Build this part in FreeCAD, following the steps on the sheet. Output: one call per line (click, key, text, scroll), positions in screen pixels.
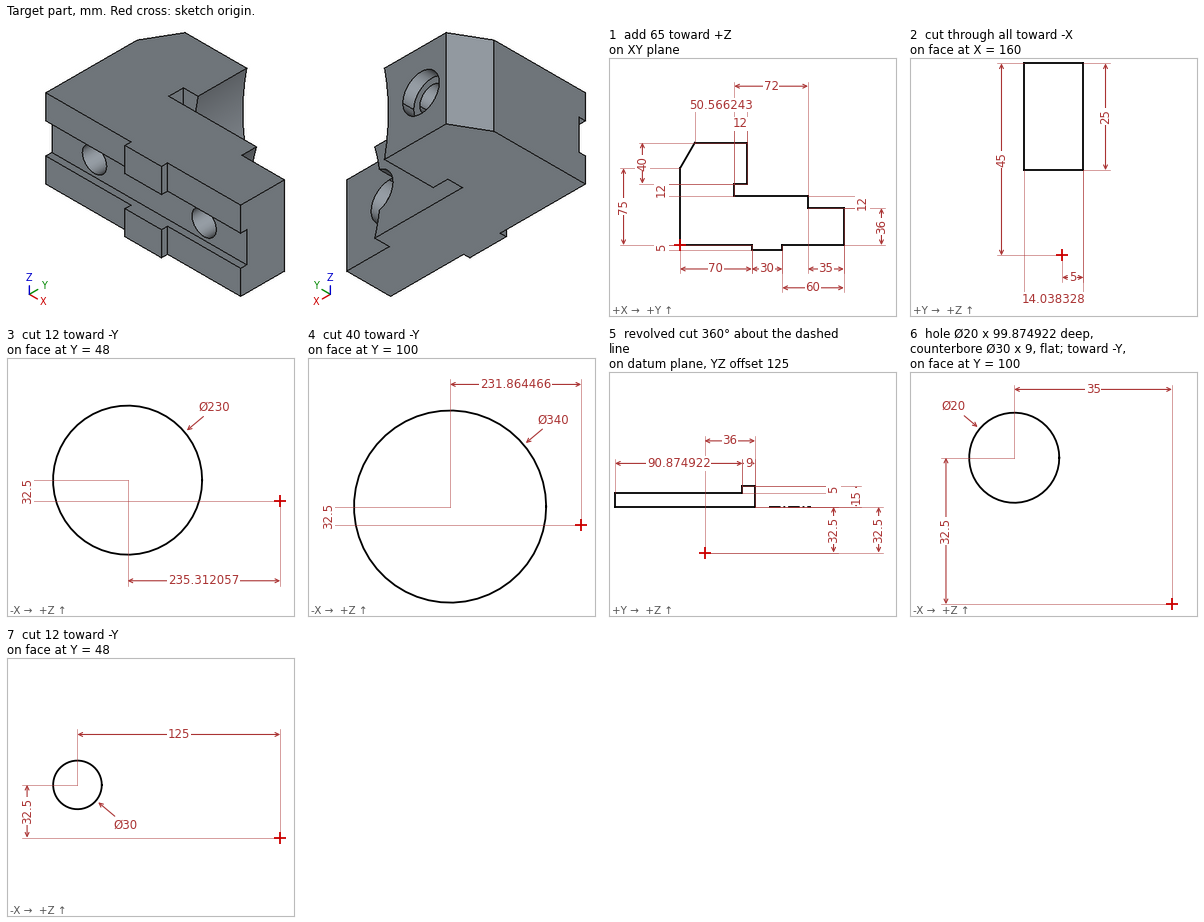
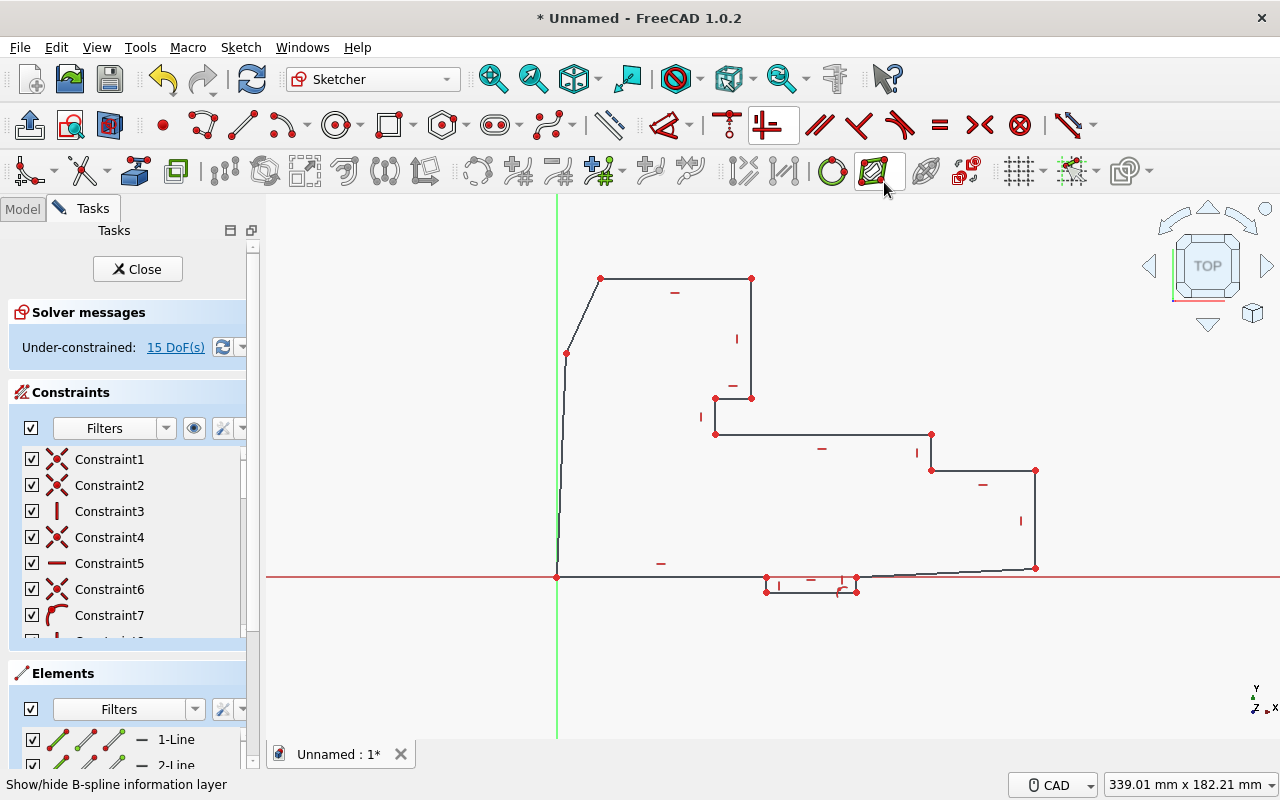
click(910, 575)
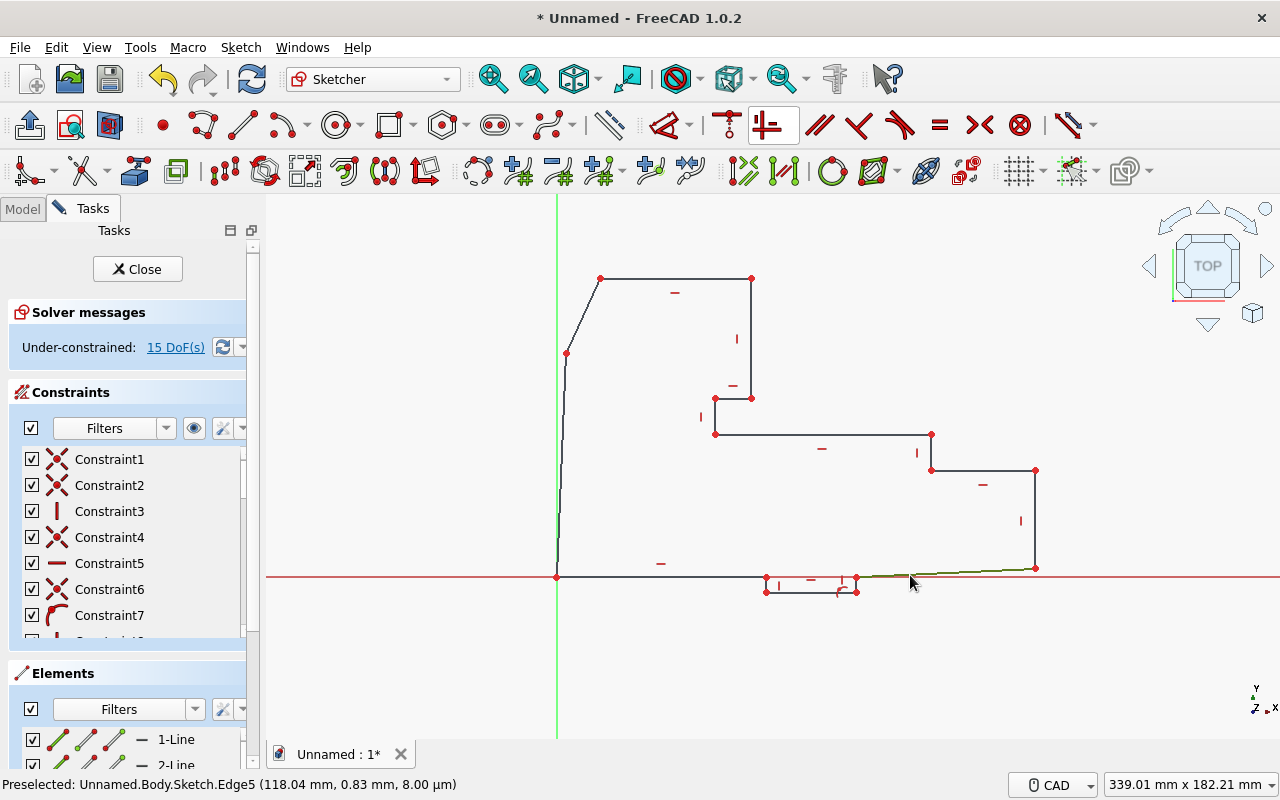
key(h)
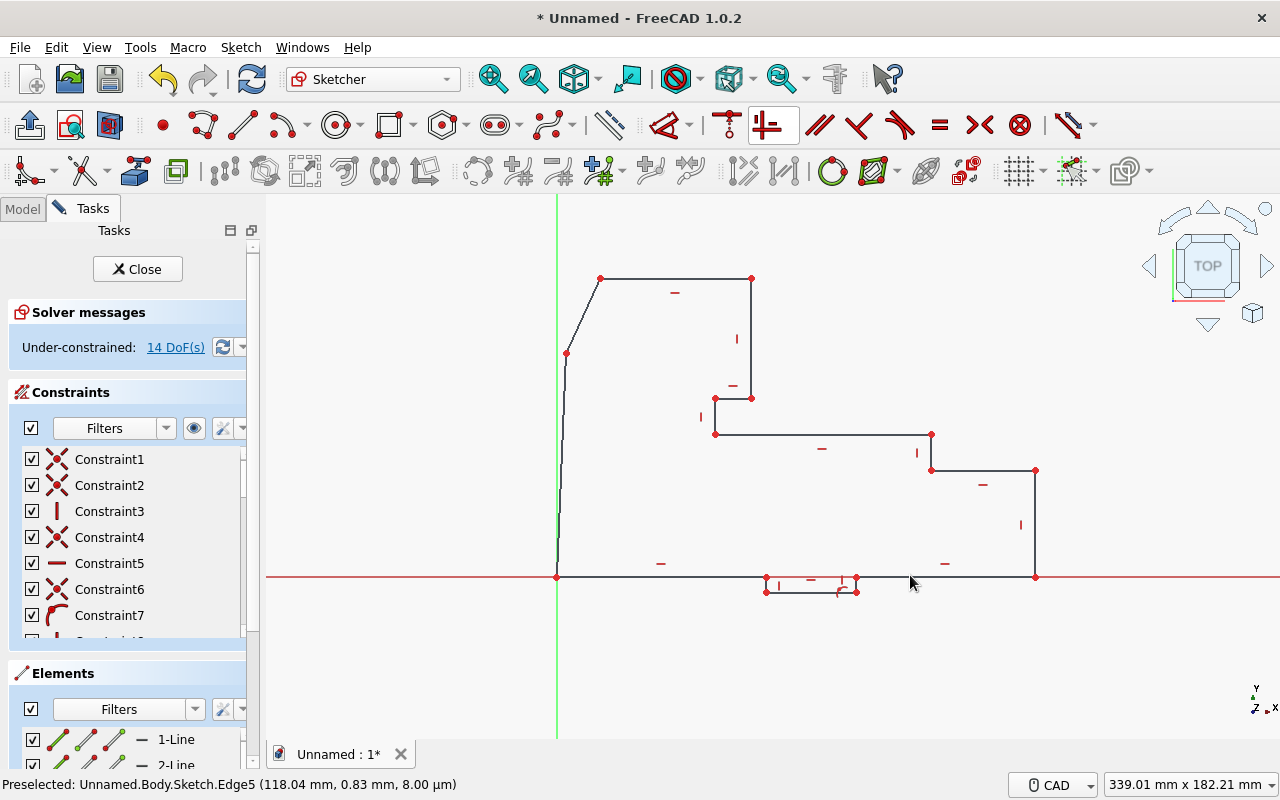
click(560, 510)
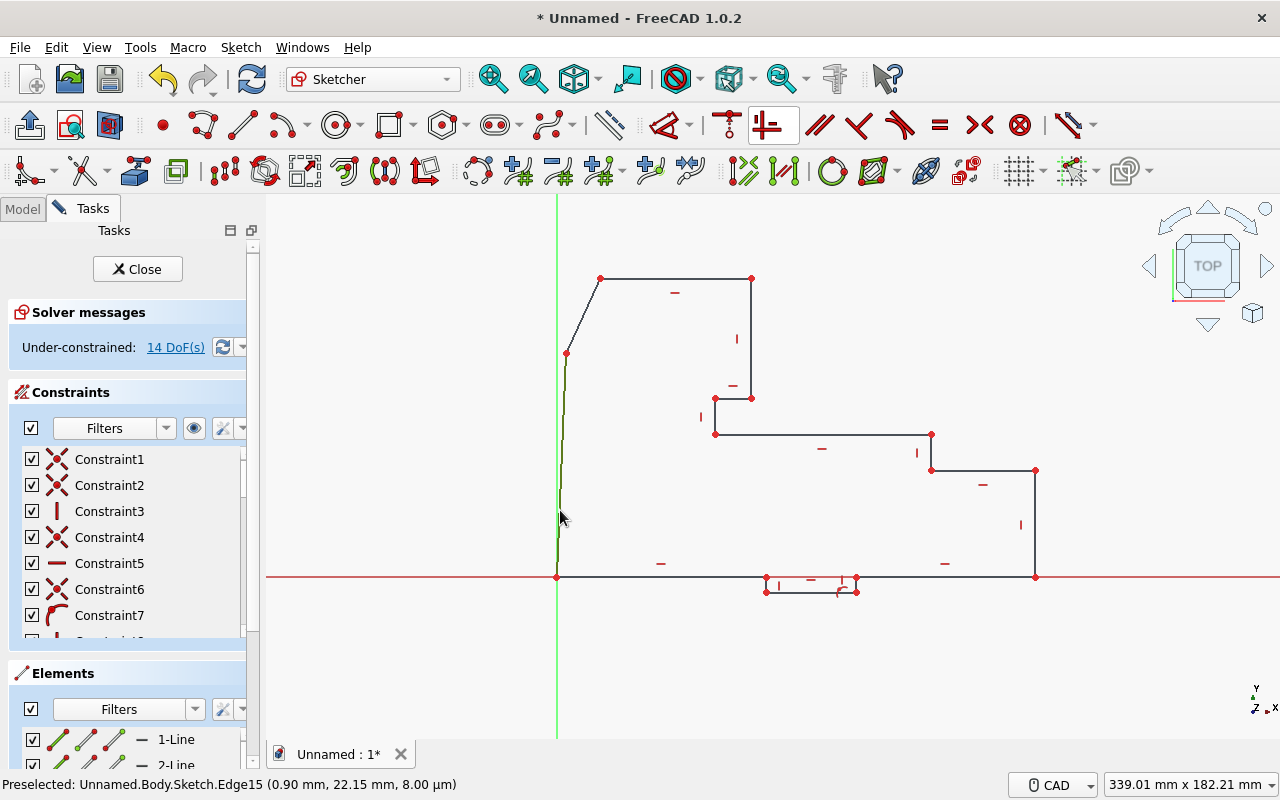
key(v)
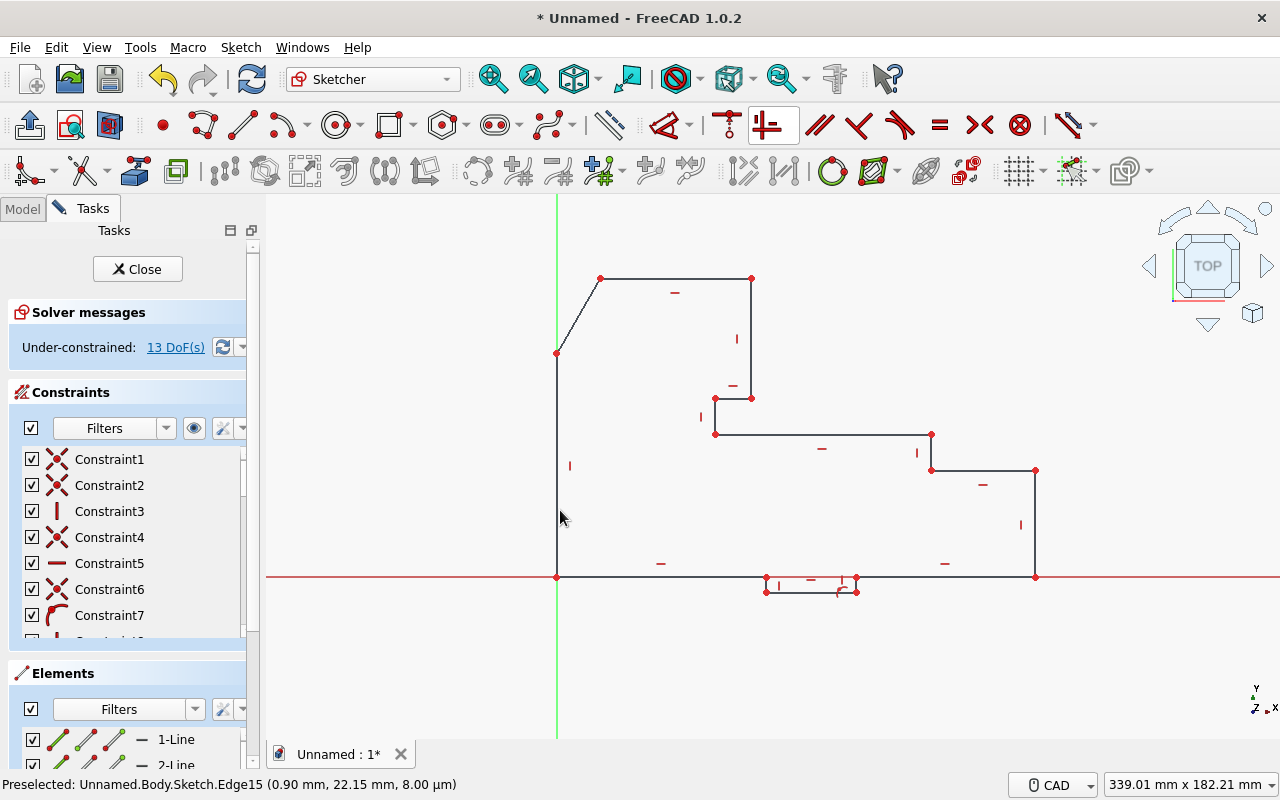
click(664, 126)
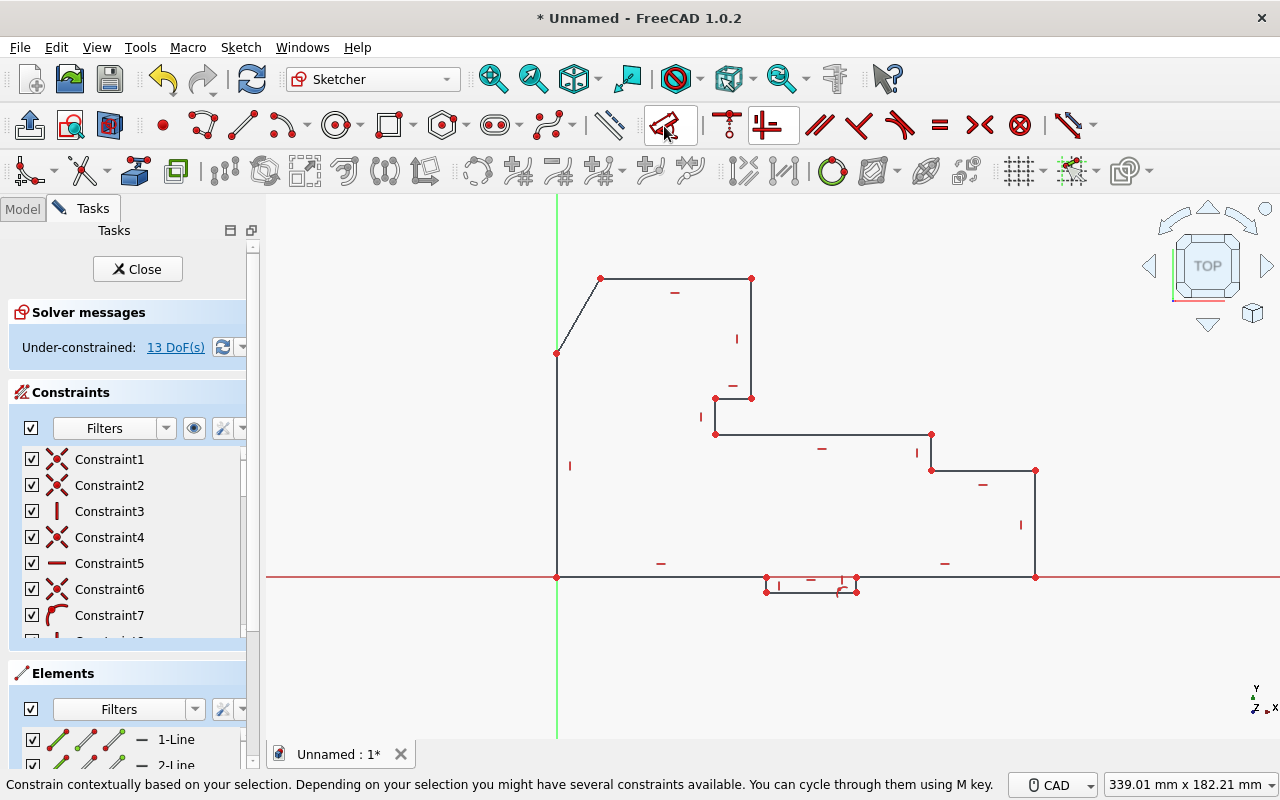
scroll(766, 585, up, 5)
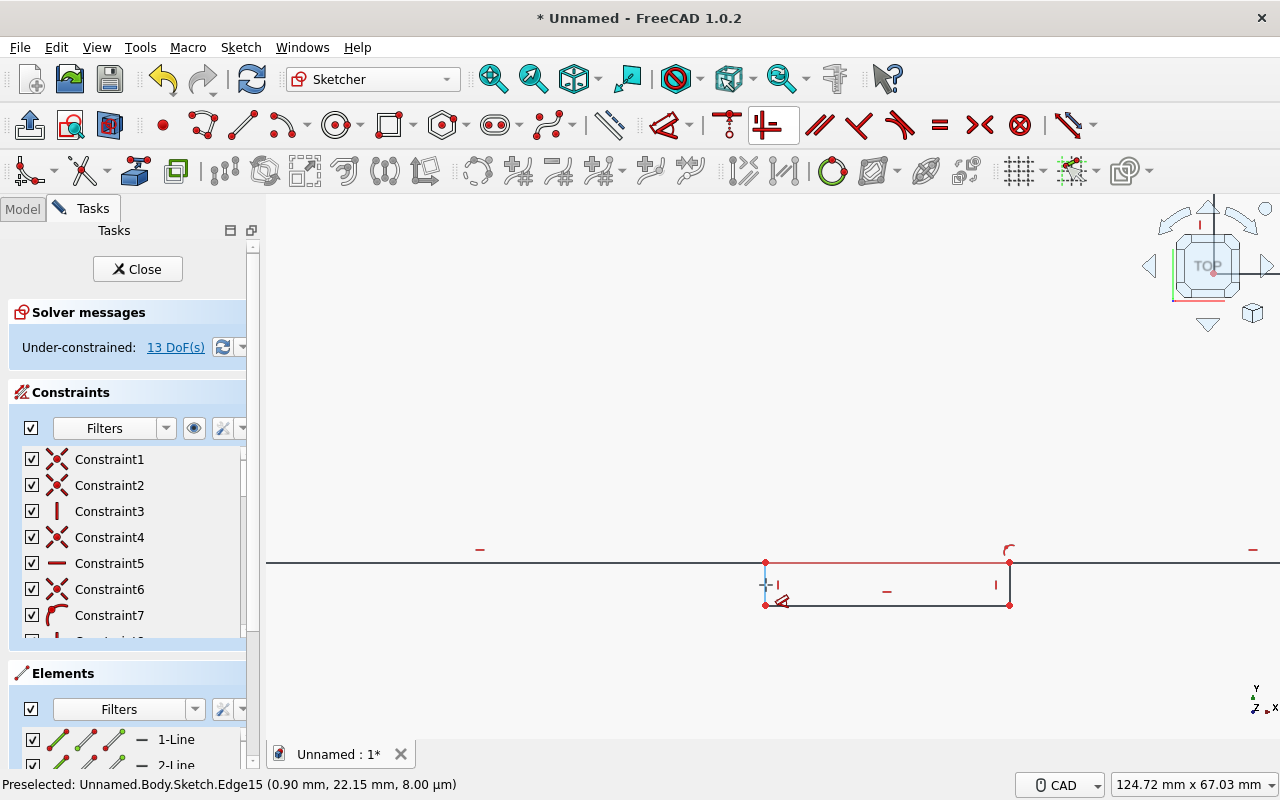
click(765, 584)
click(731, 584)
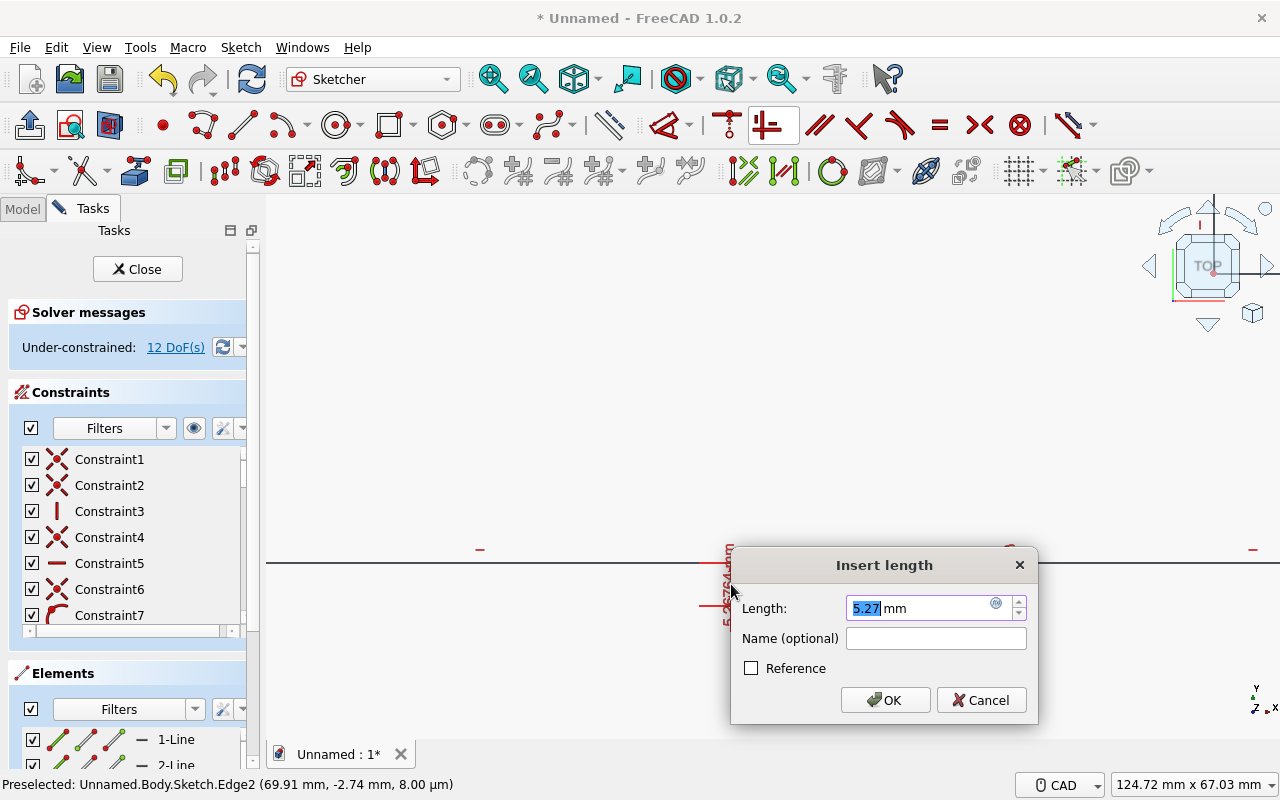
text(5)
key(Return)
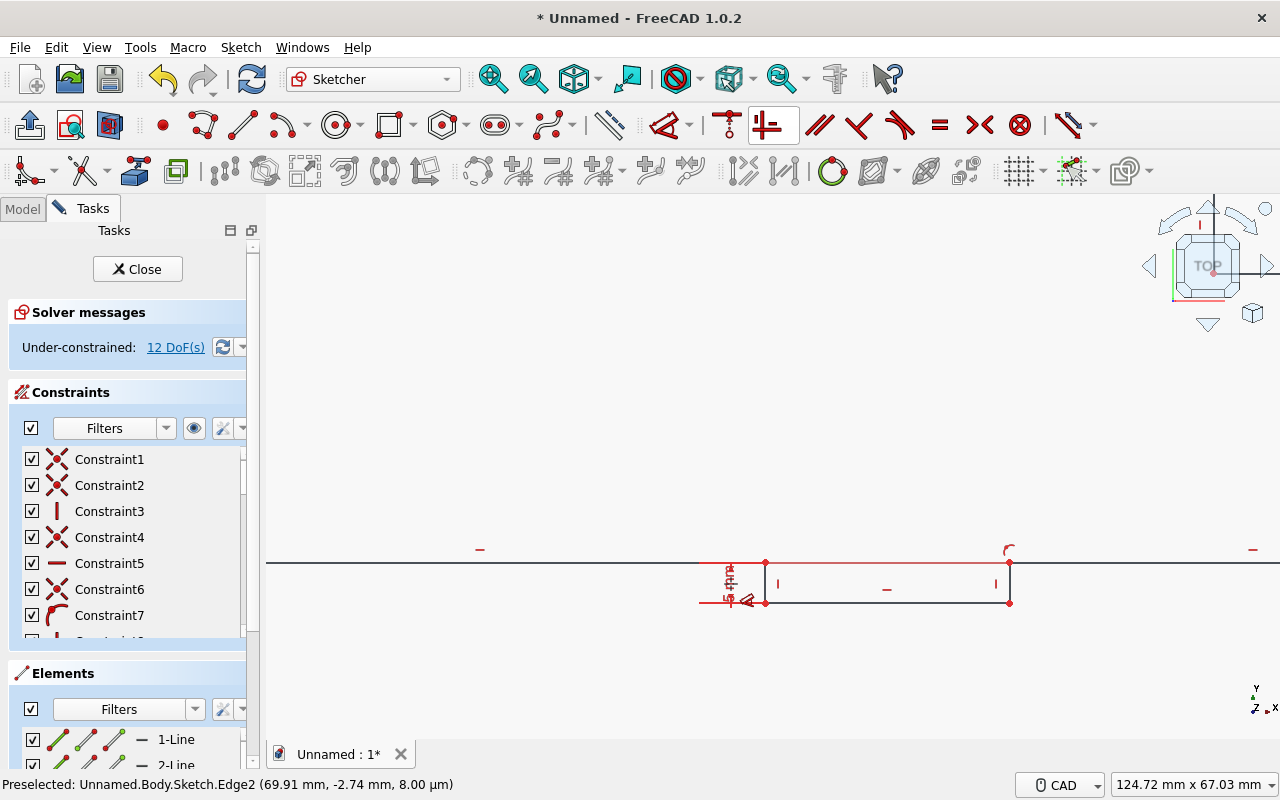
click(367, 563)
click(530, 597)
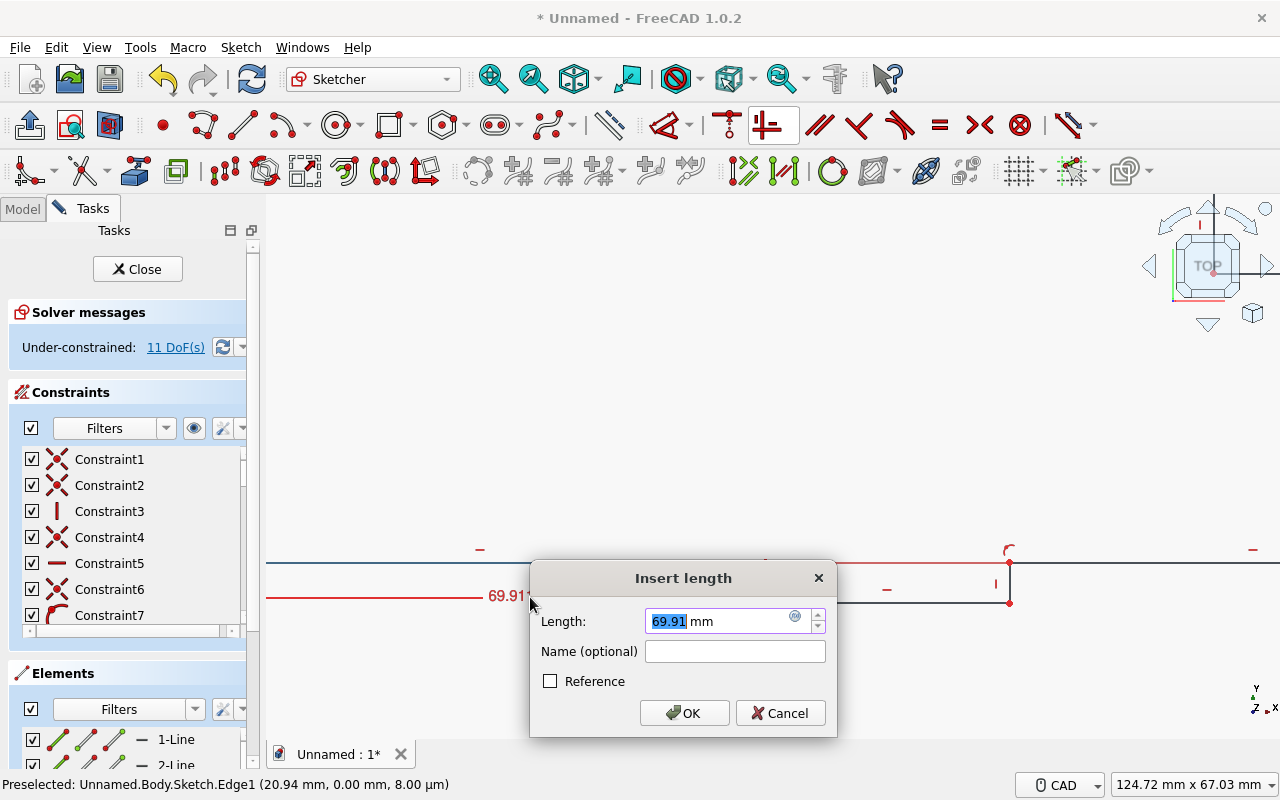
text(70)
key(Return)